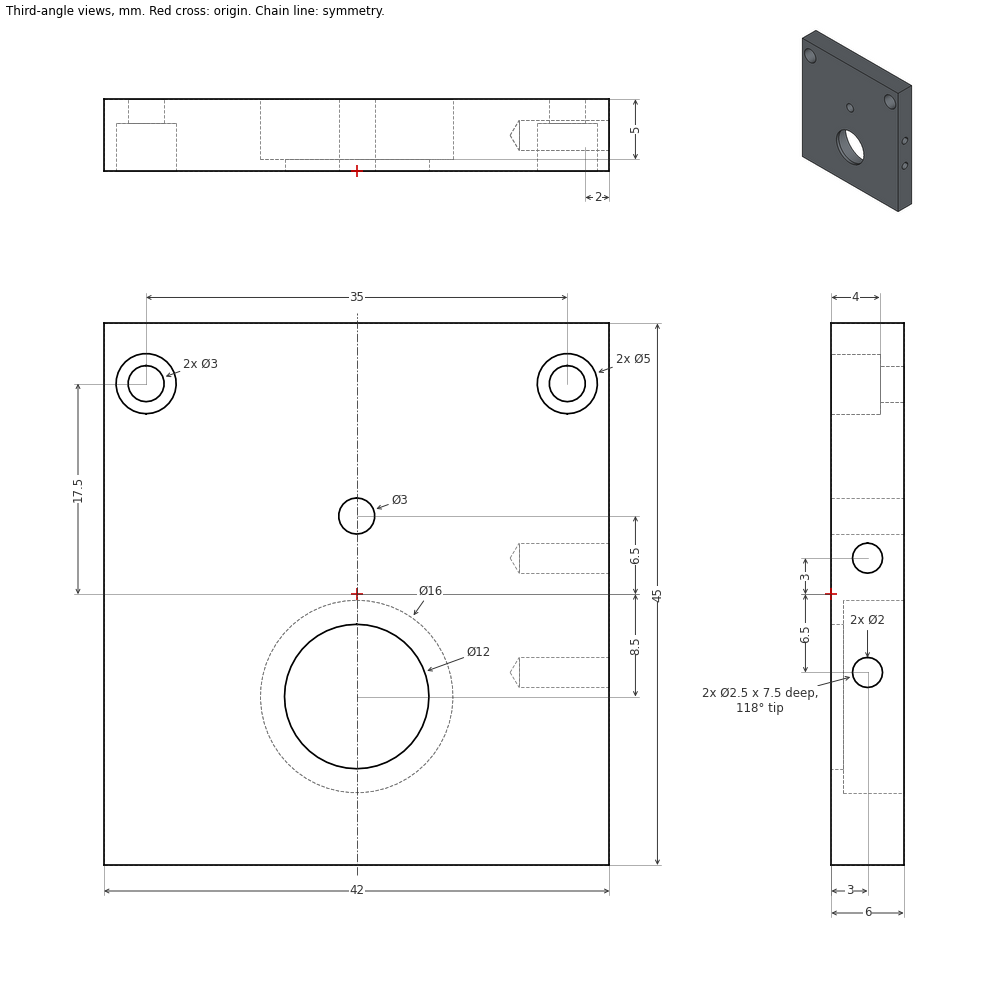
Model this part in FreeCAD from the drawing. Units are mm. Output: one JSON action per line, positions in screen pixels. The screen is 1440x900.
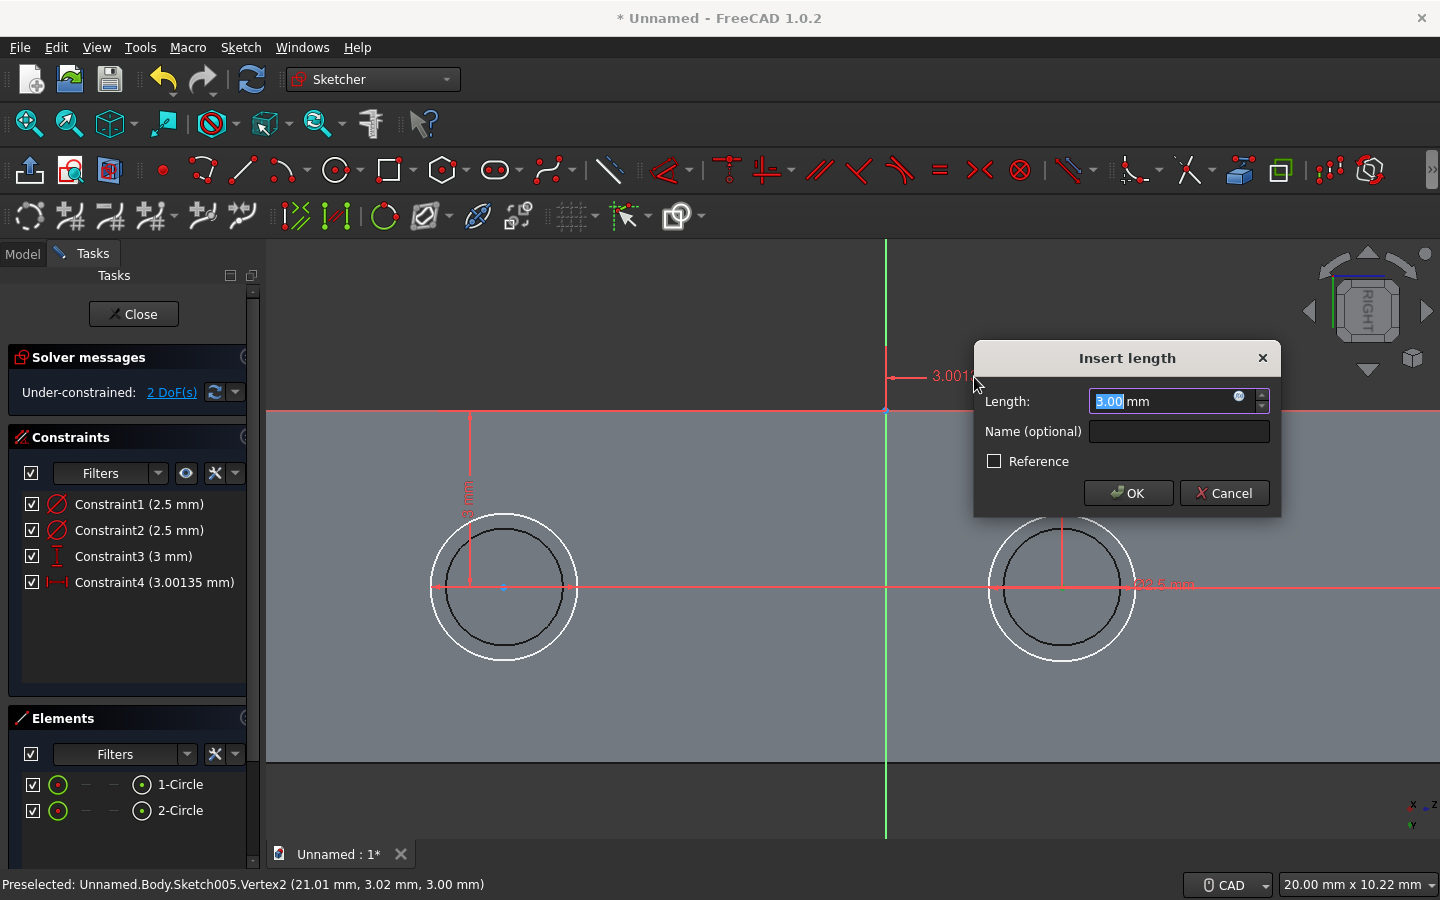
{"action": "type", "text": "3"}
{"action": "key", "text": "Return"}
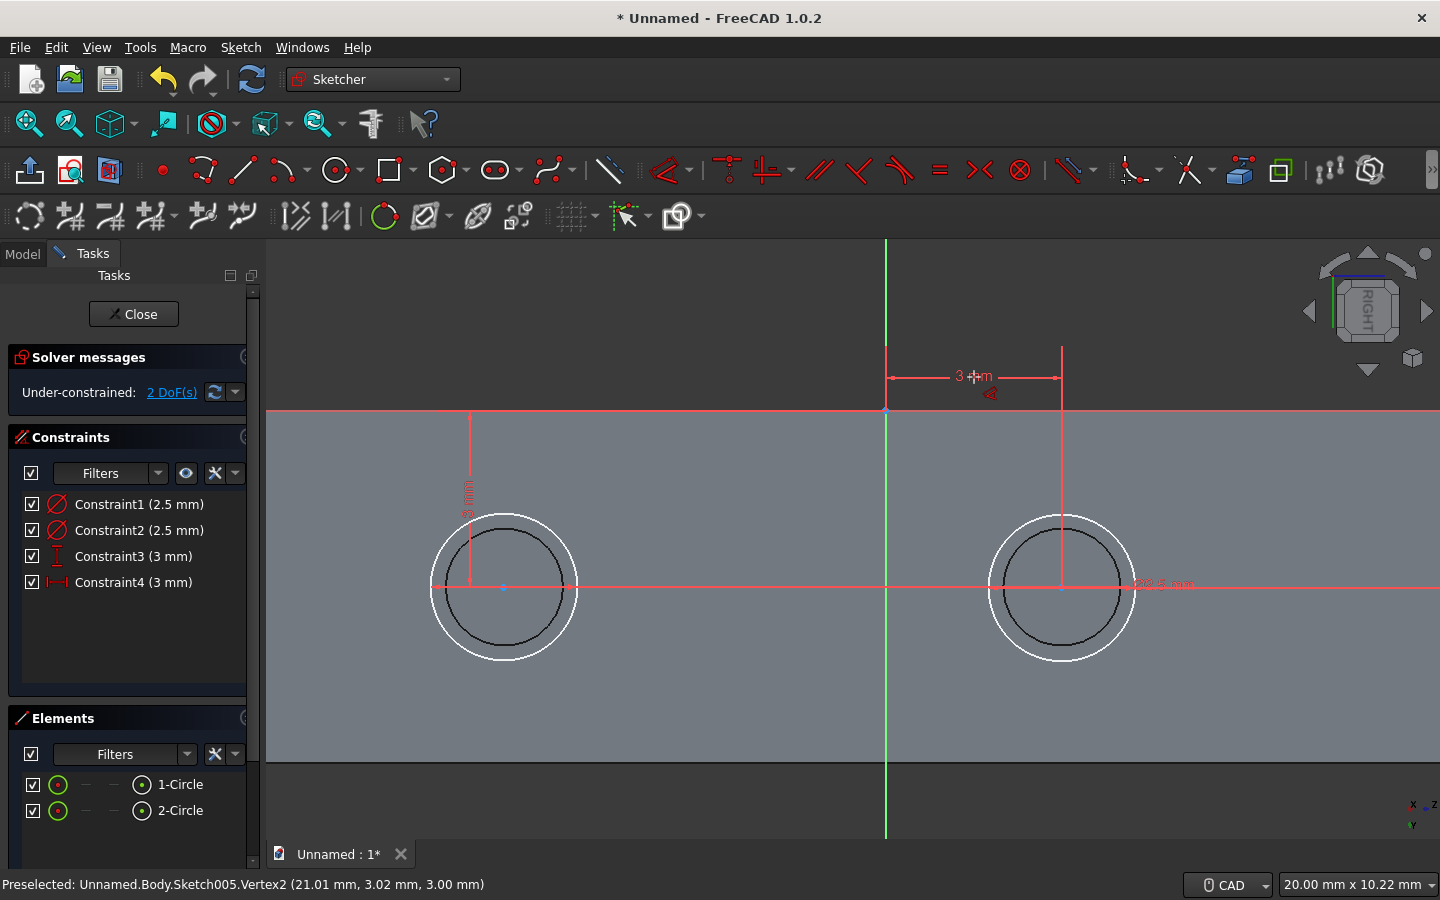
{"action": "left_click", "coordinate": [1062, 588]}
{"action": "left_click", "coordinate": [1096, 499]}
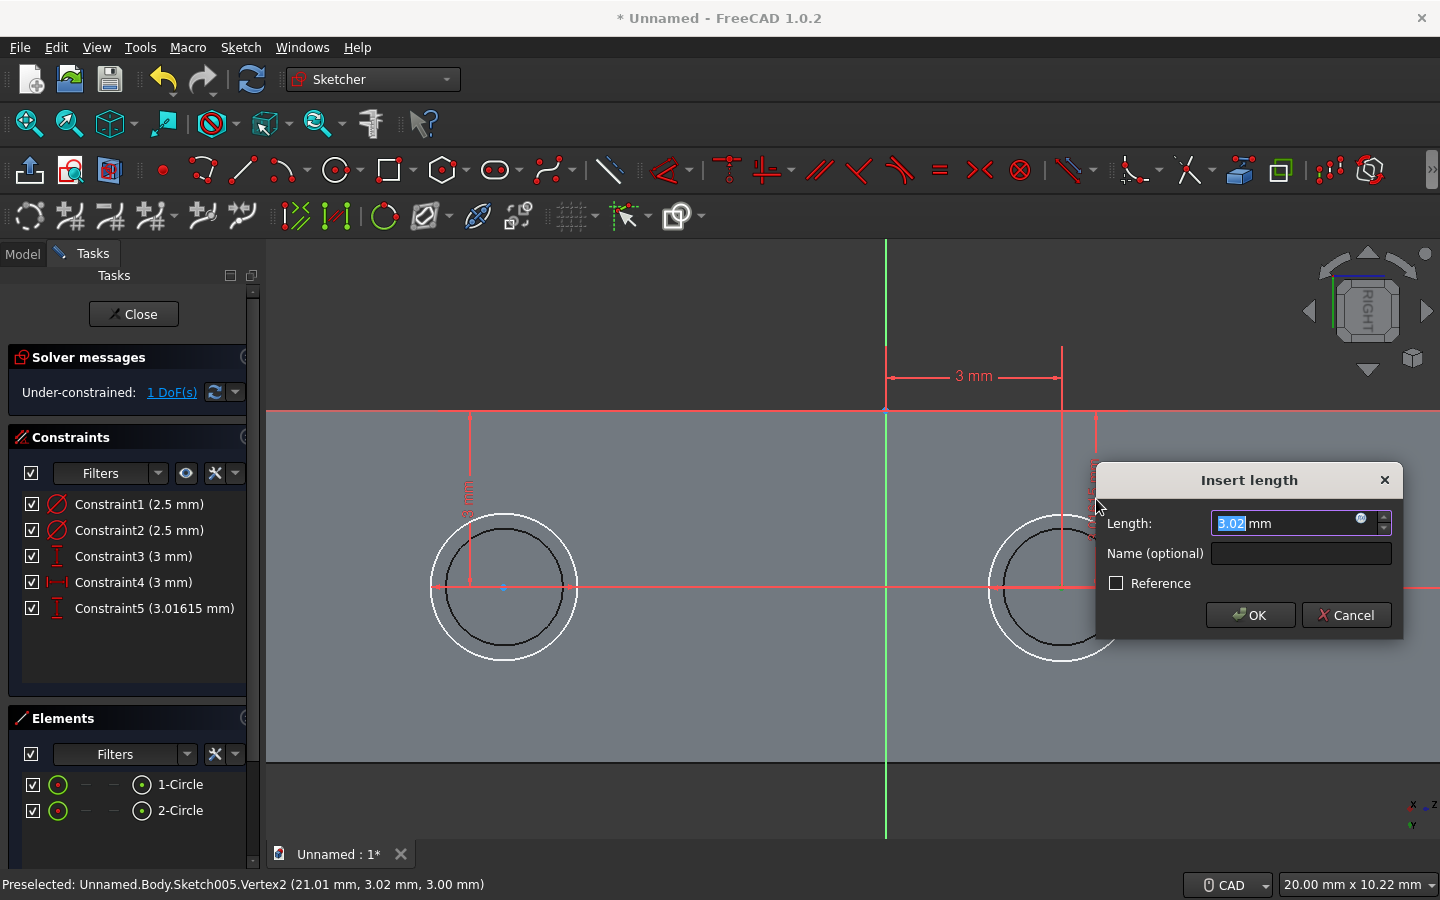
{"action": "type", "text": "3"}
{"action": "key", "text": "Return"}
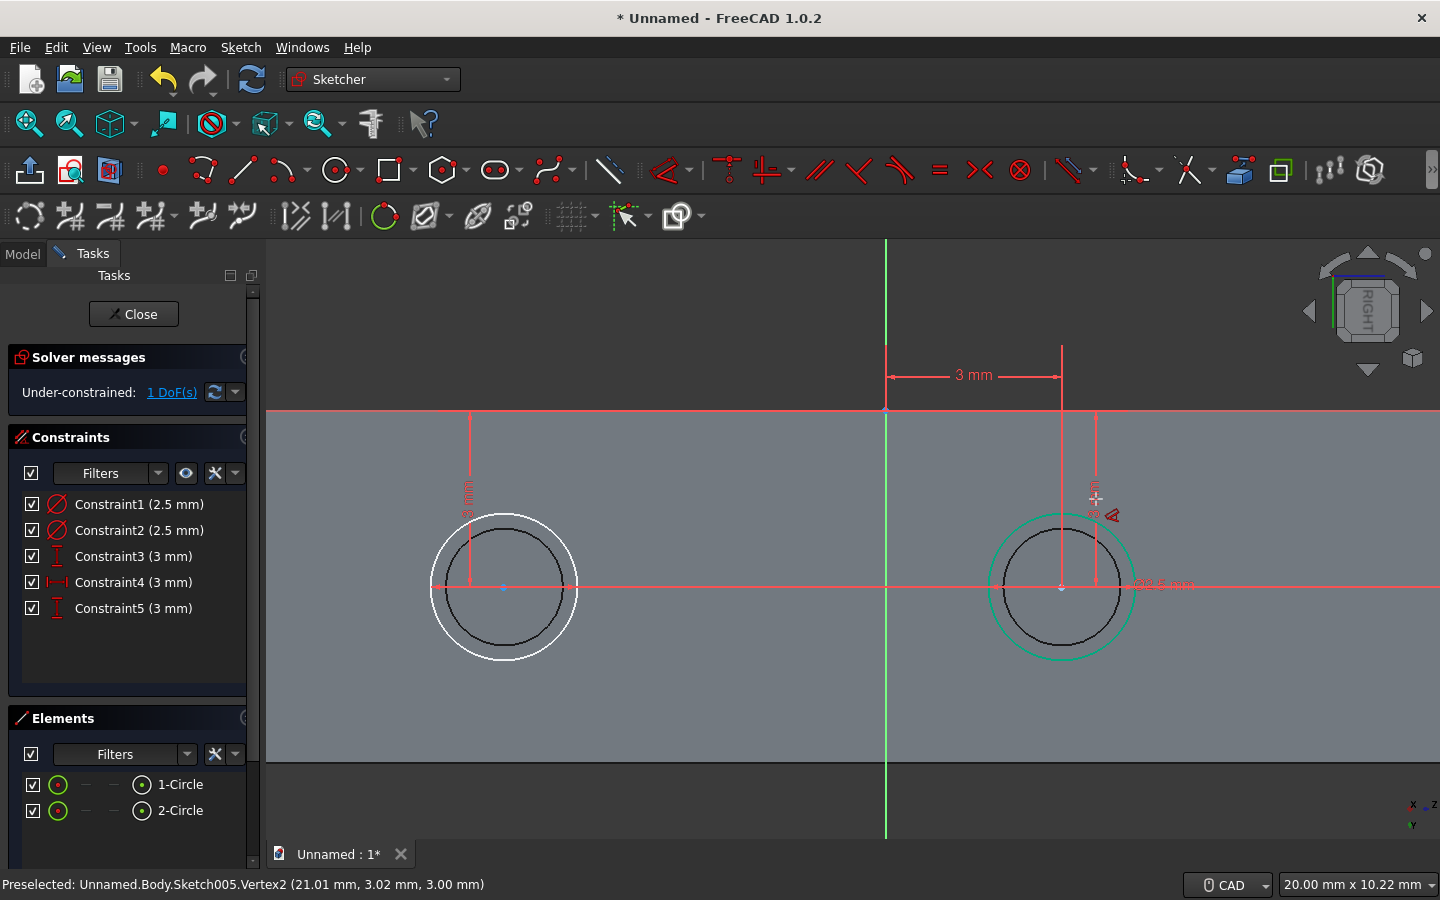
{"action": "left_click", "coordinate": [504, 587]}
{"action": "left_click", "coordinate": [695, 377]}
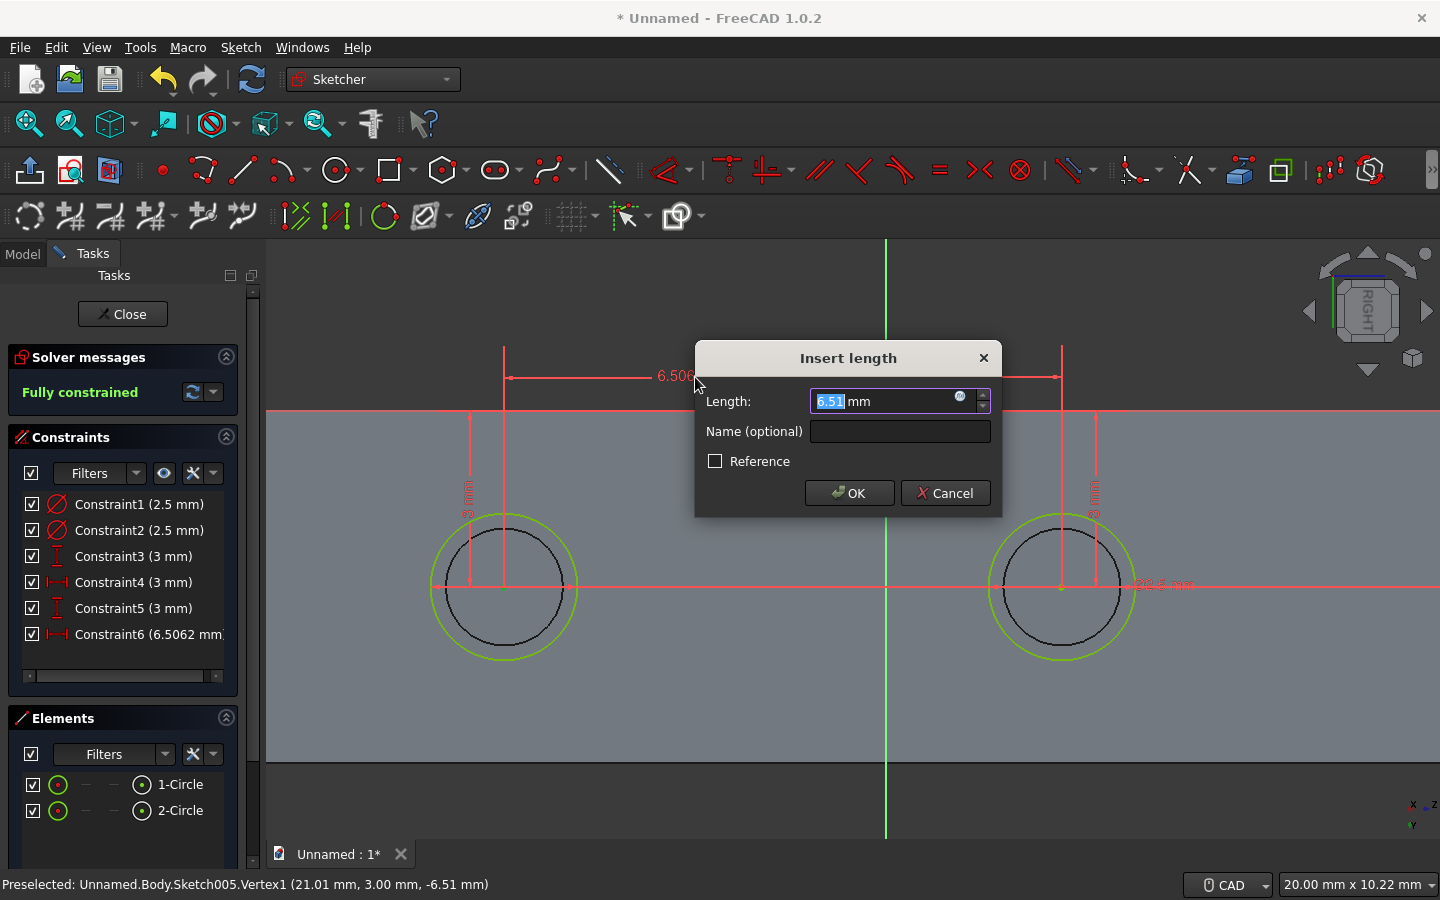
{"action": "type", "text": "6.5"}
{"action": "key", "text": "Return"}
{"action": "key", "text": "Escape"}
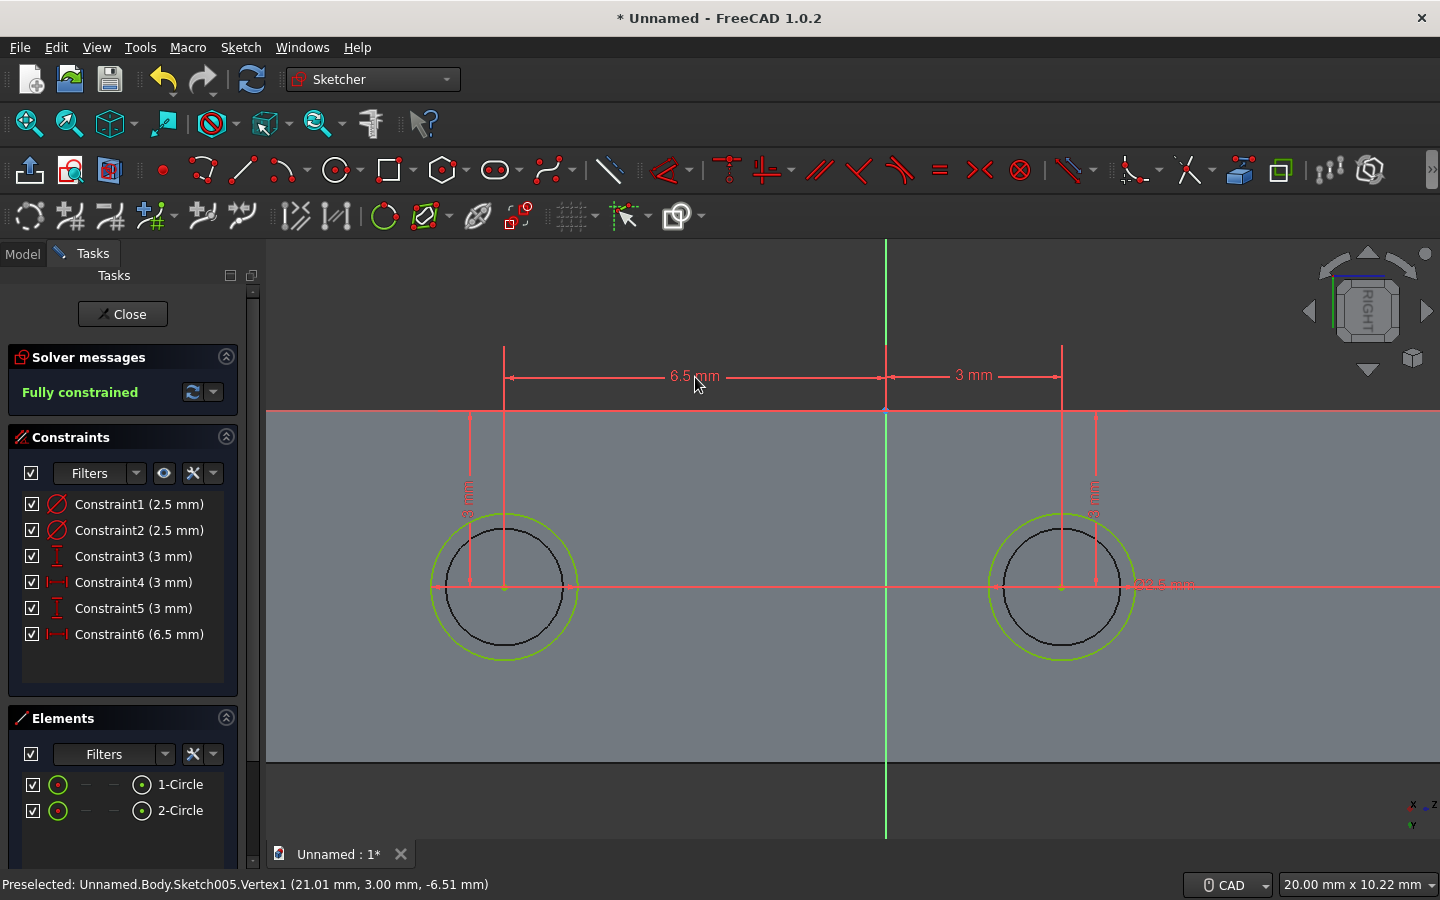
{"action": "left_click", "coordinate": [123, 314]}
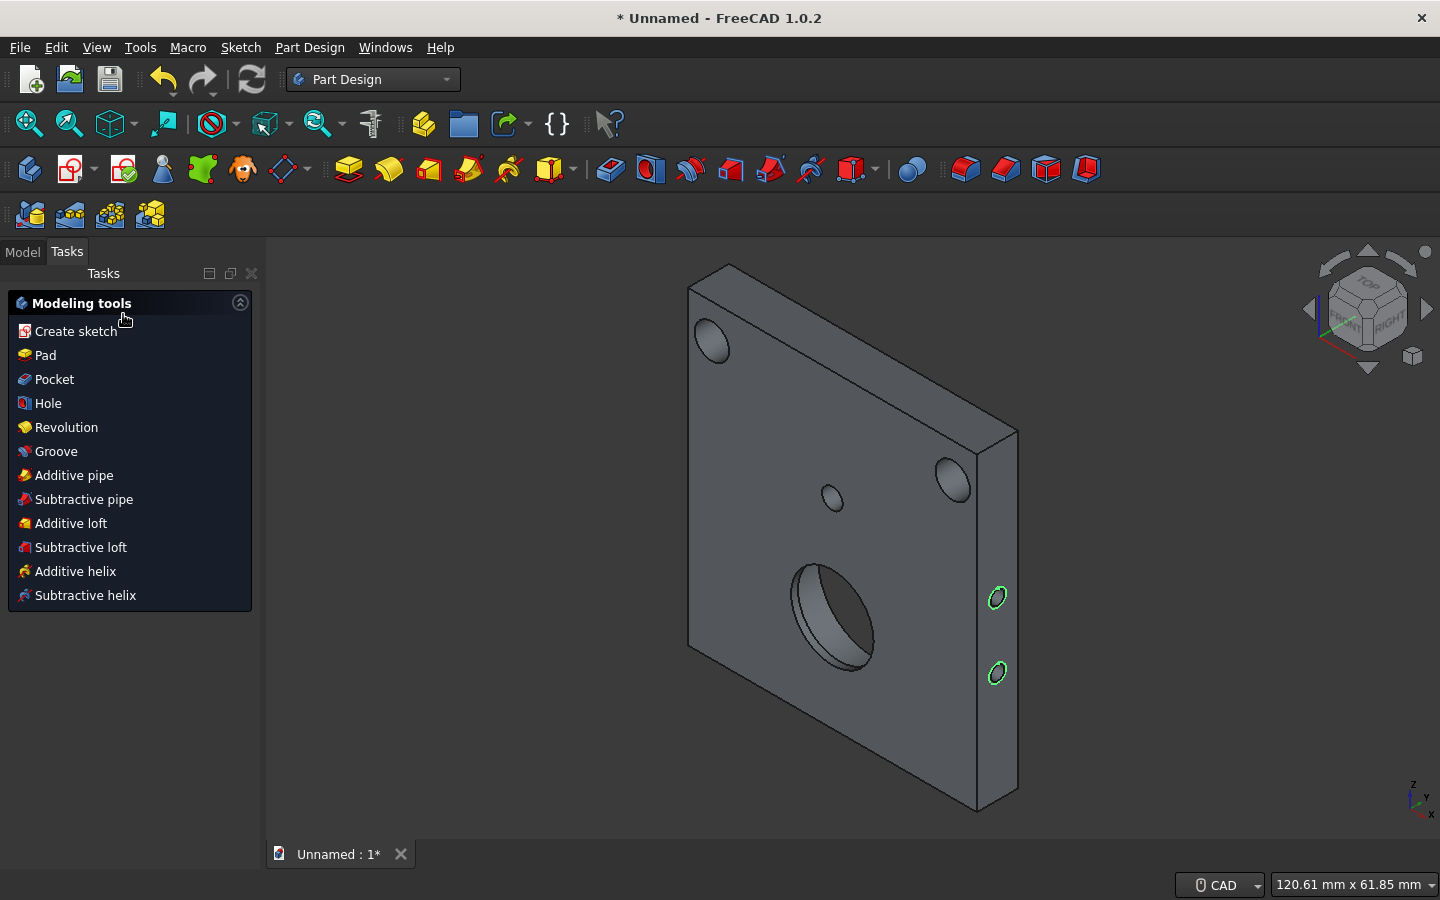
{"action": "left_click", "coordinate": [652, 170]}